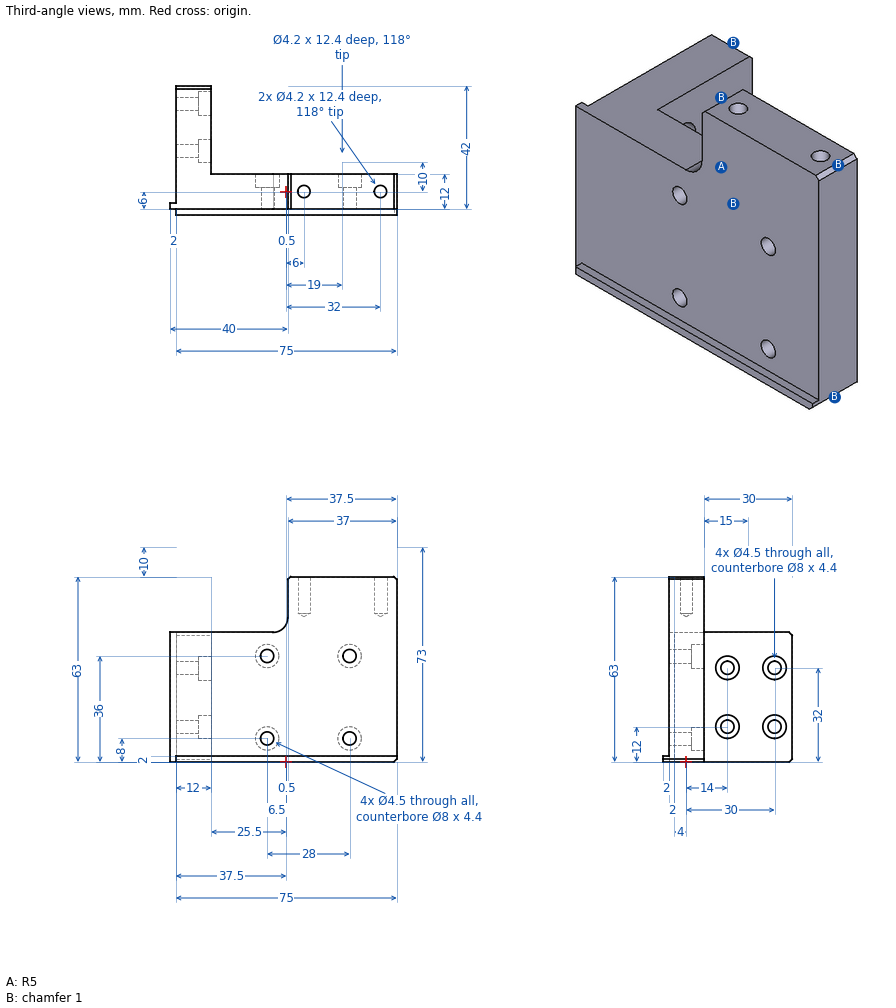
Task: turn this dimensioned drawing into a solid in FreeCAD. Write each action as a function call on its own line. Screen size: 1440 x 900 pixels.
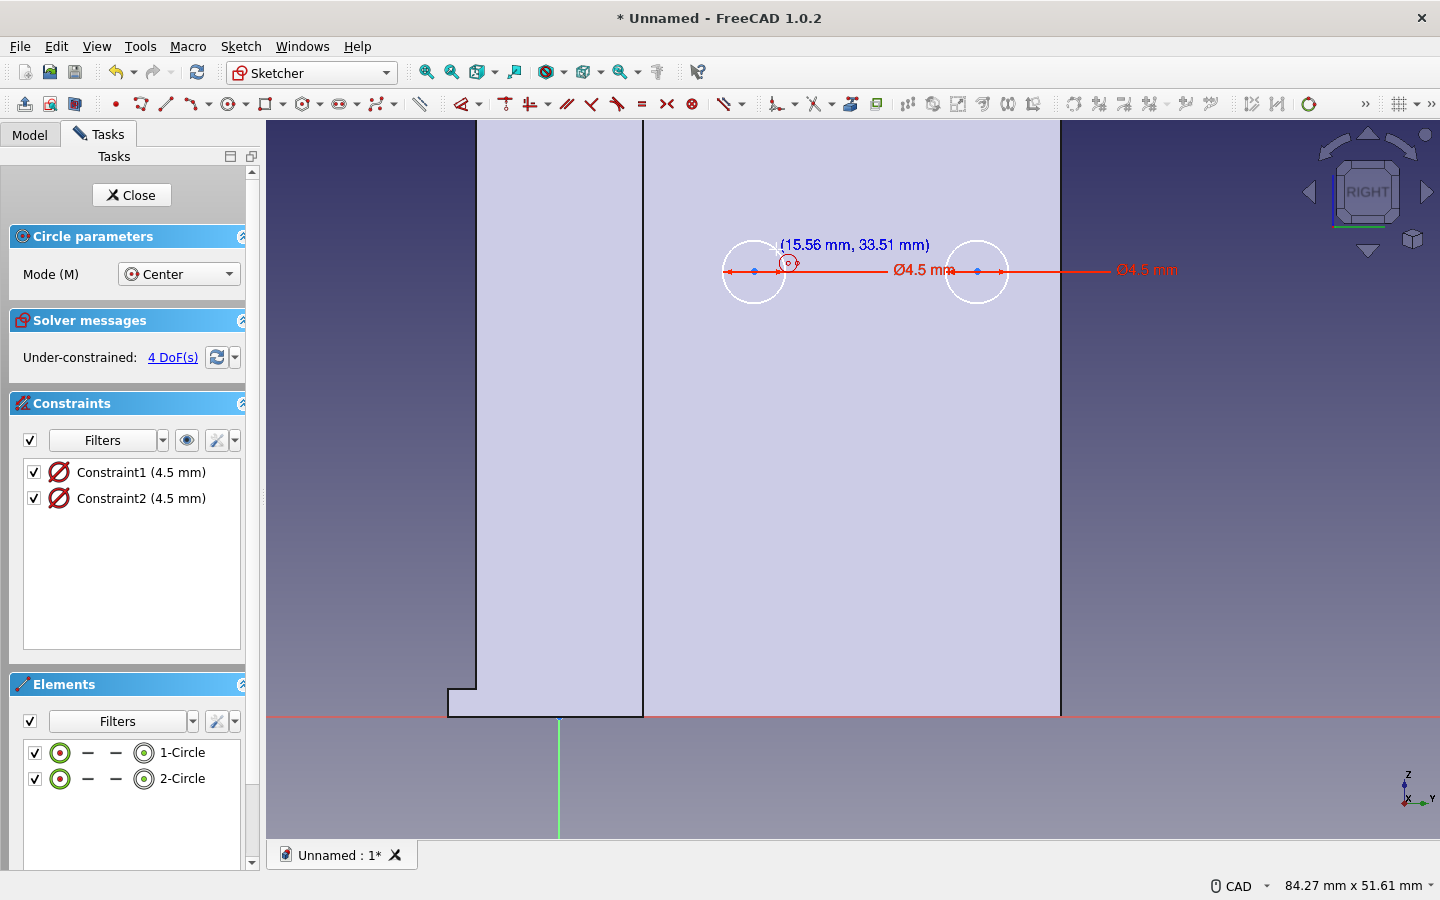
click(754, 550)
move(776, 527)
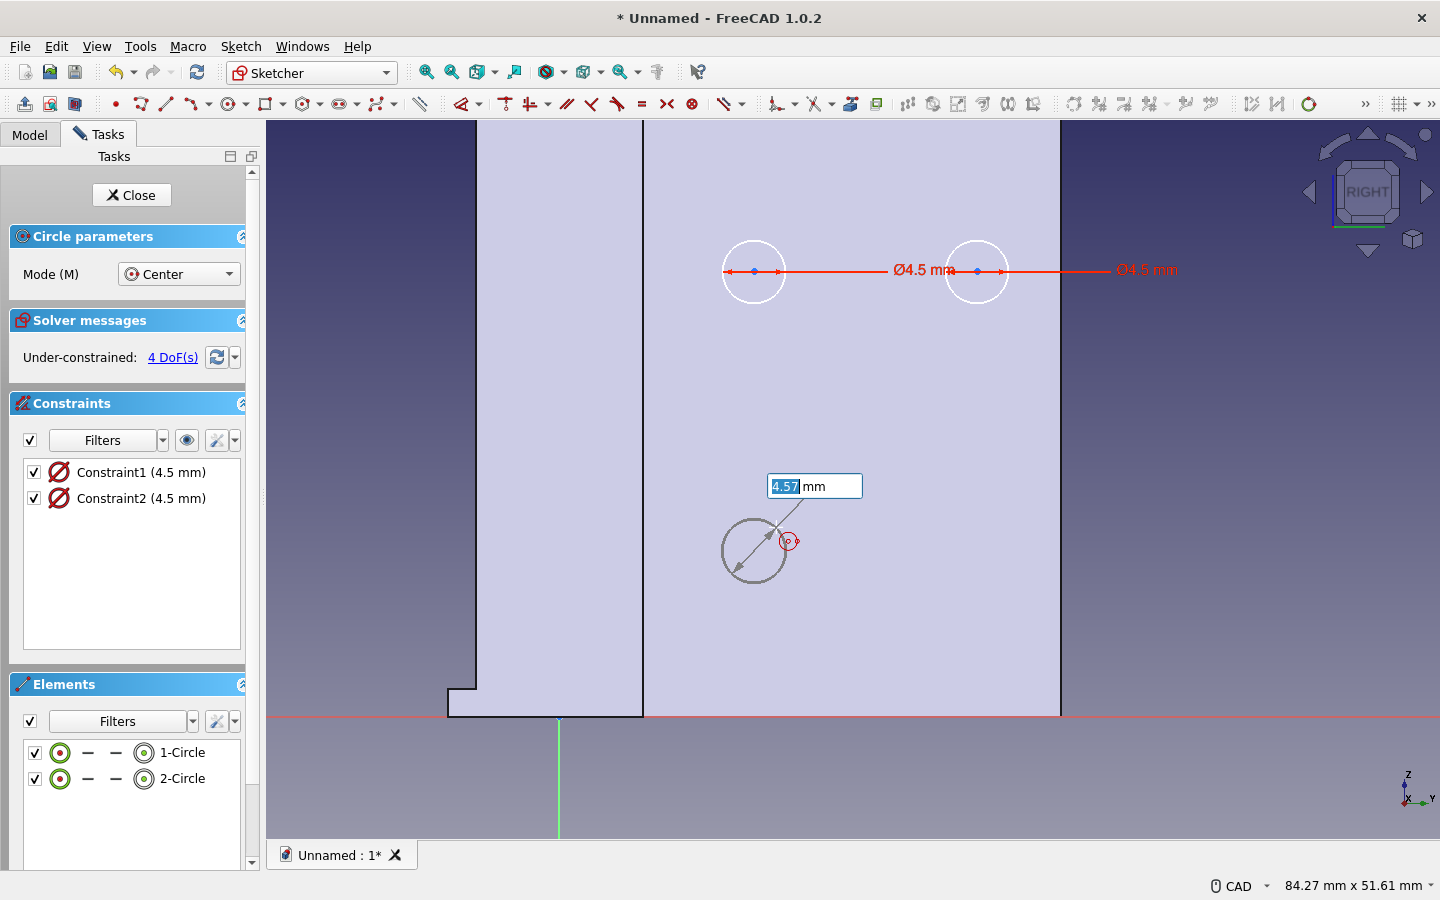
text(4.5)
key(Return)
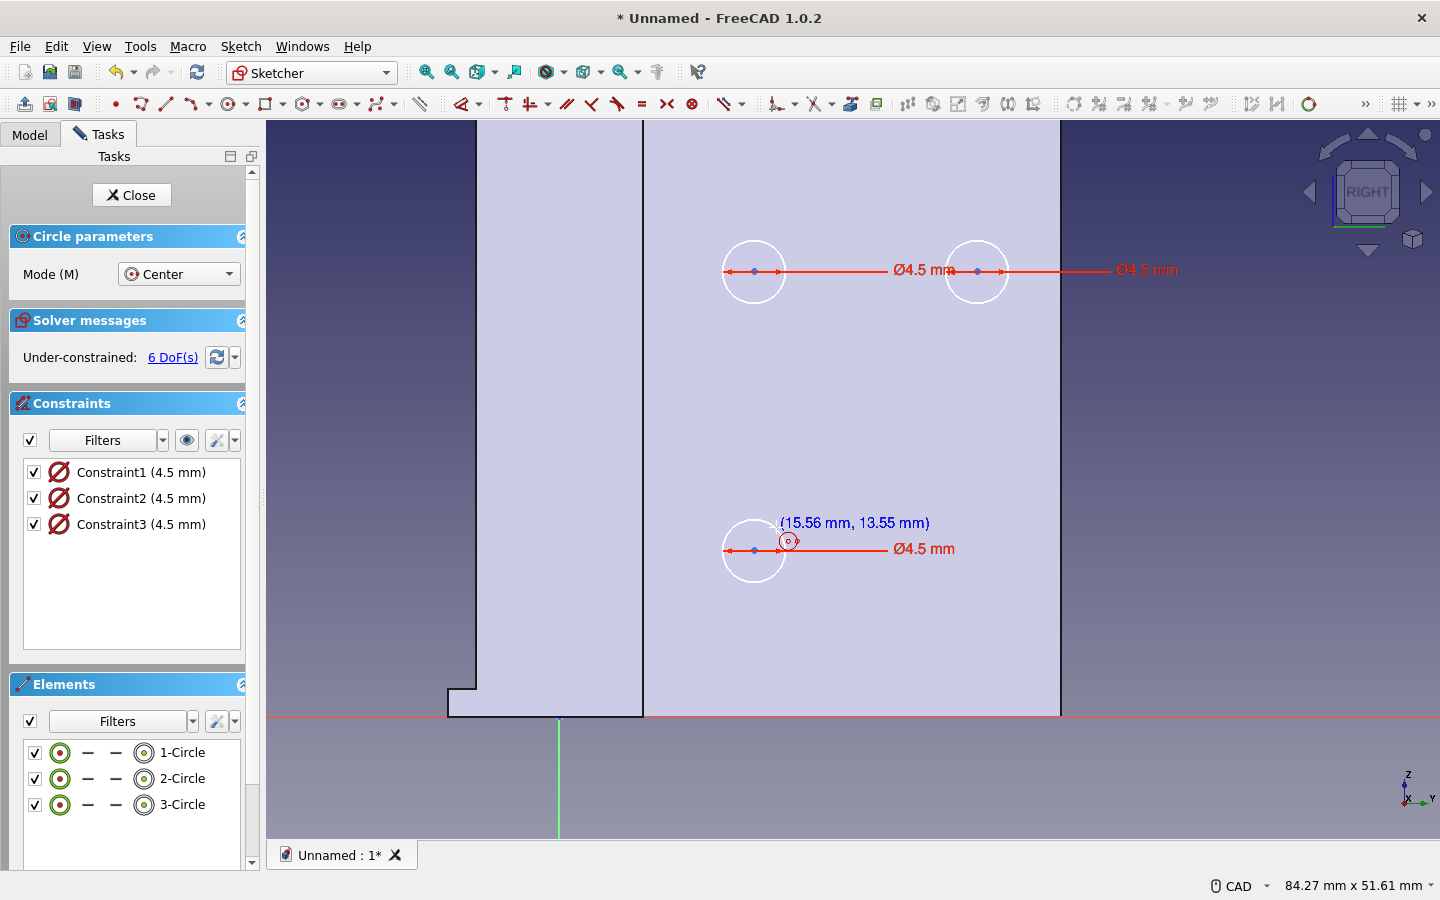
click(977, 550)
move(999, 527)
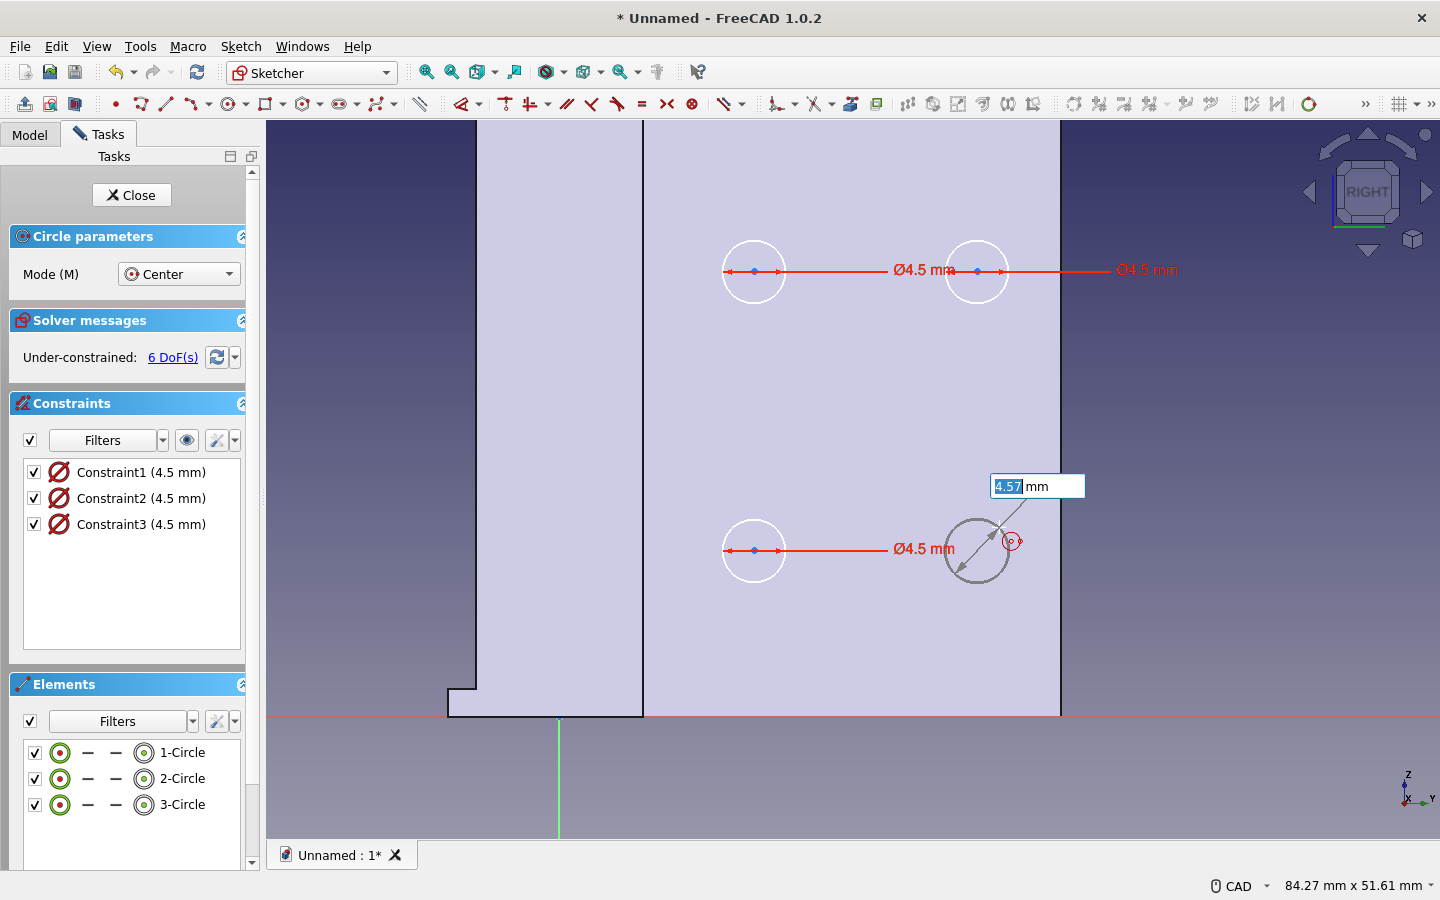
text(4.5)
key(Return)
key(Escape)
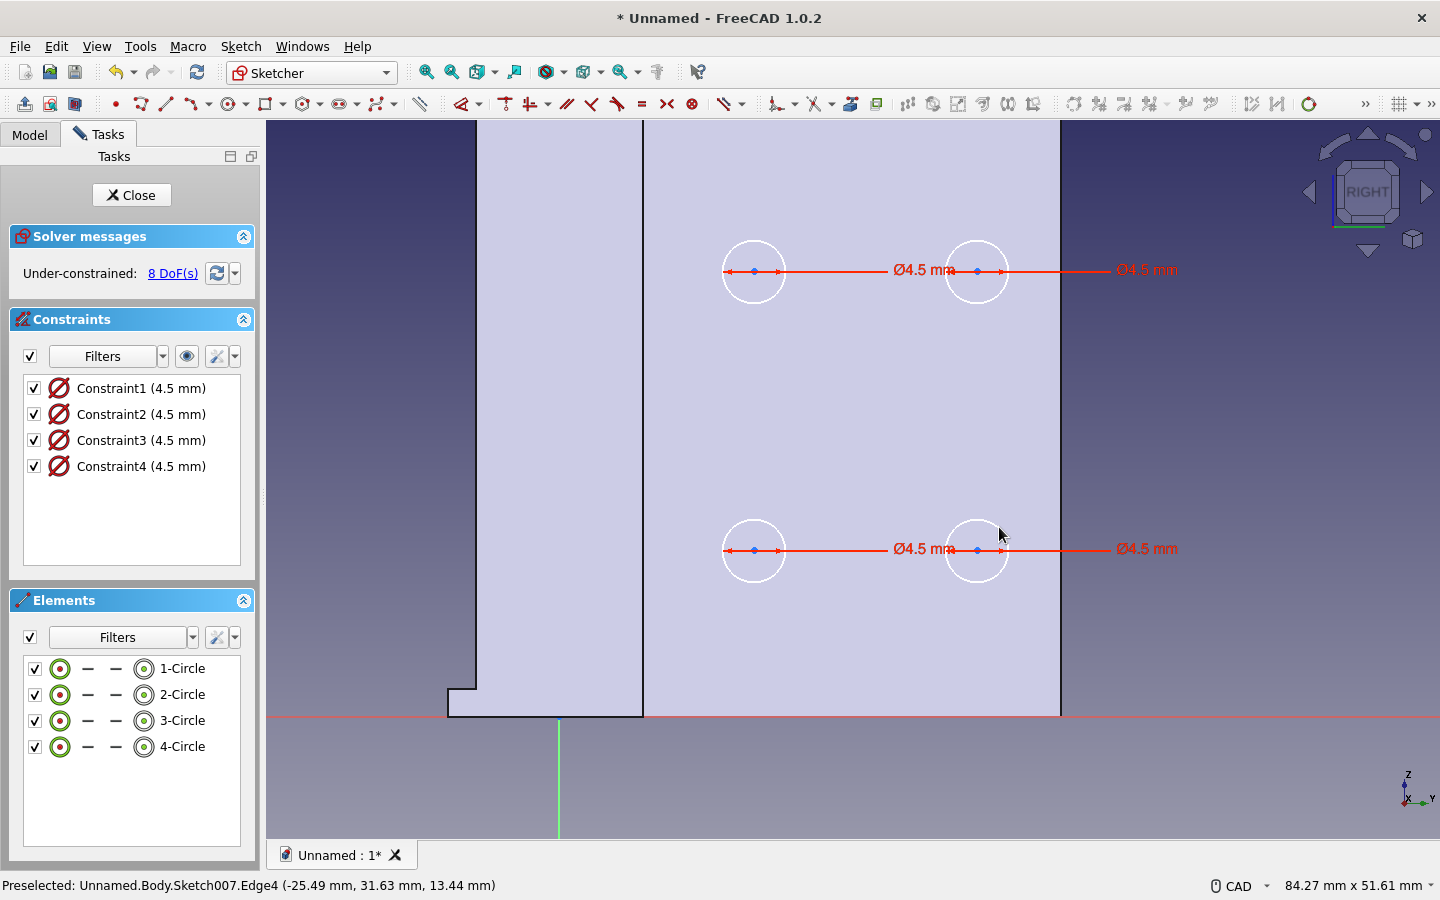
click(977, 272)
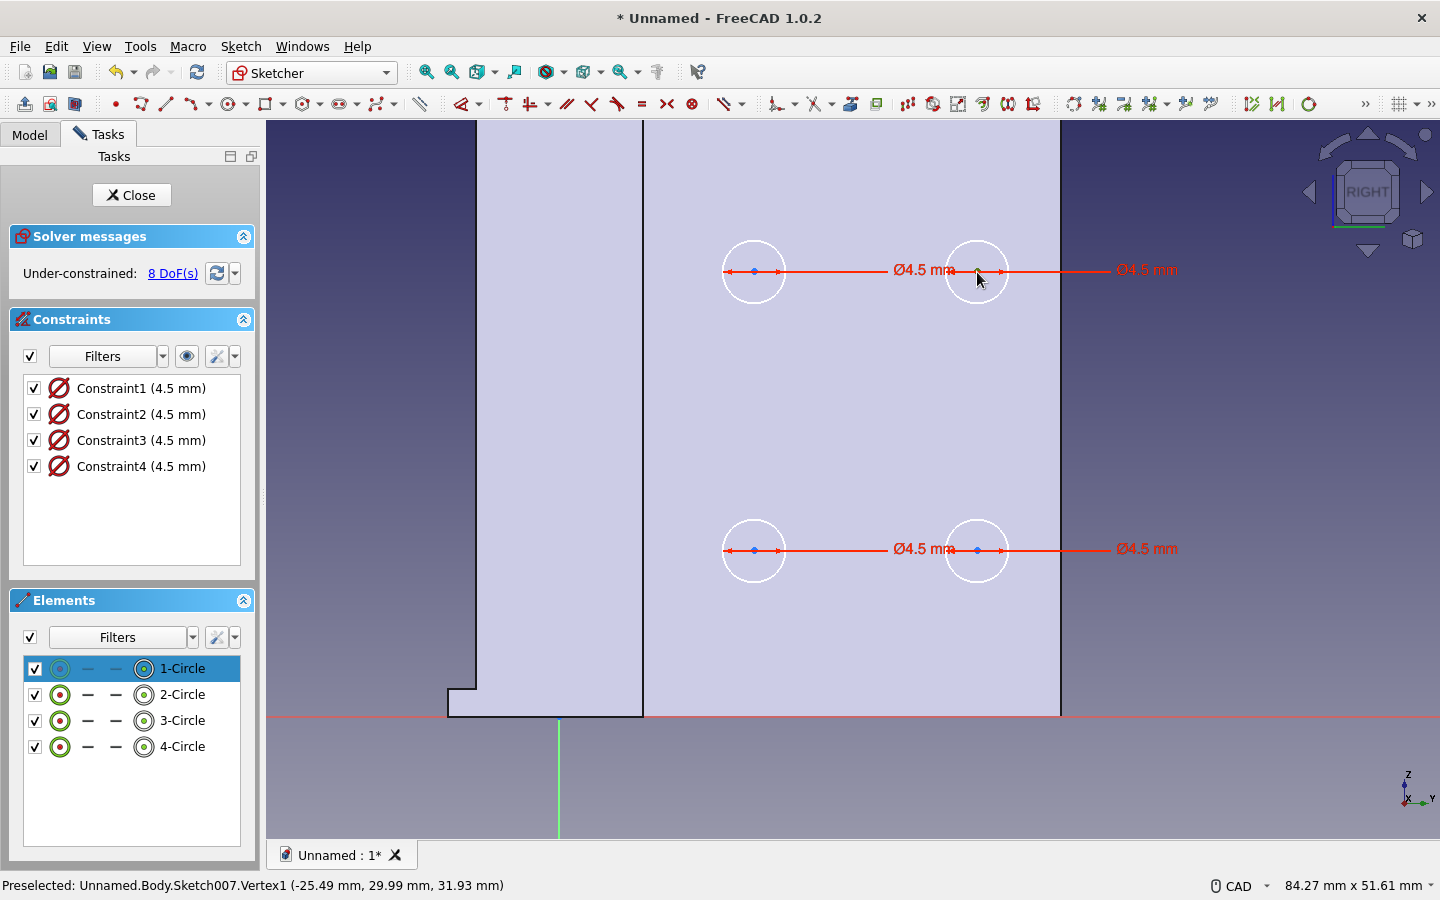
click(754, 272)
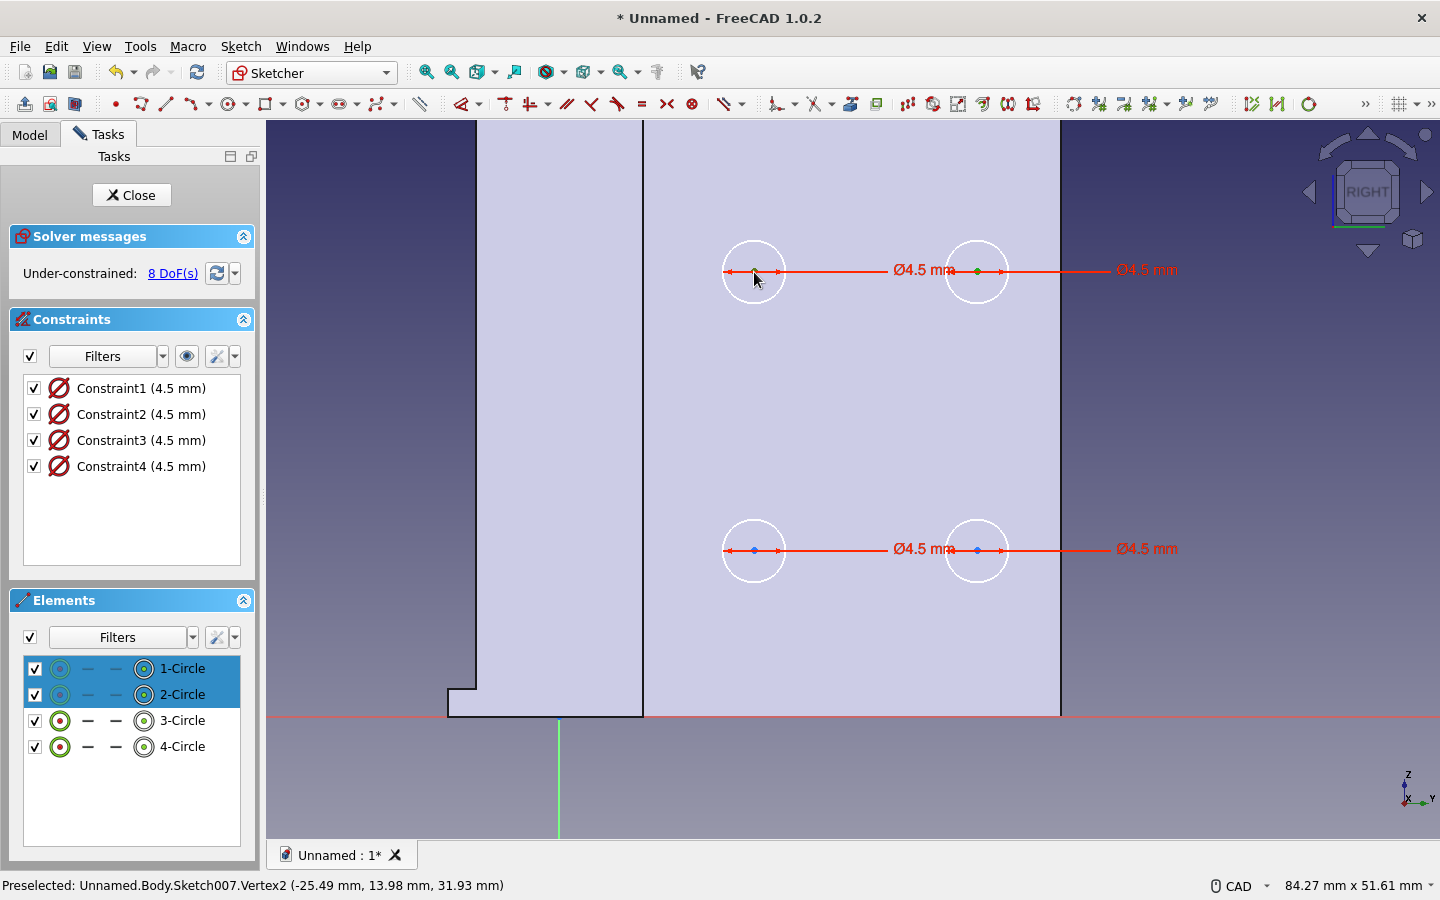
click(548, 104)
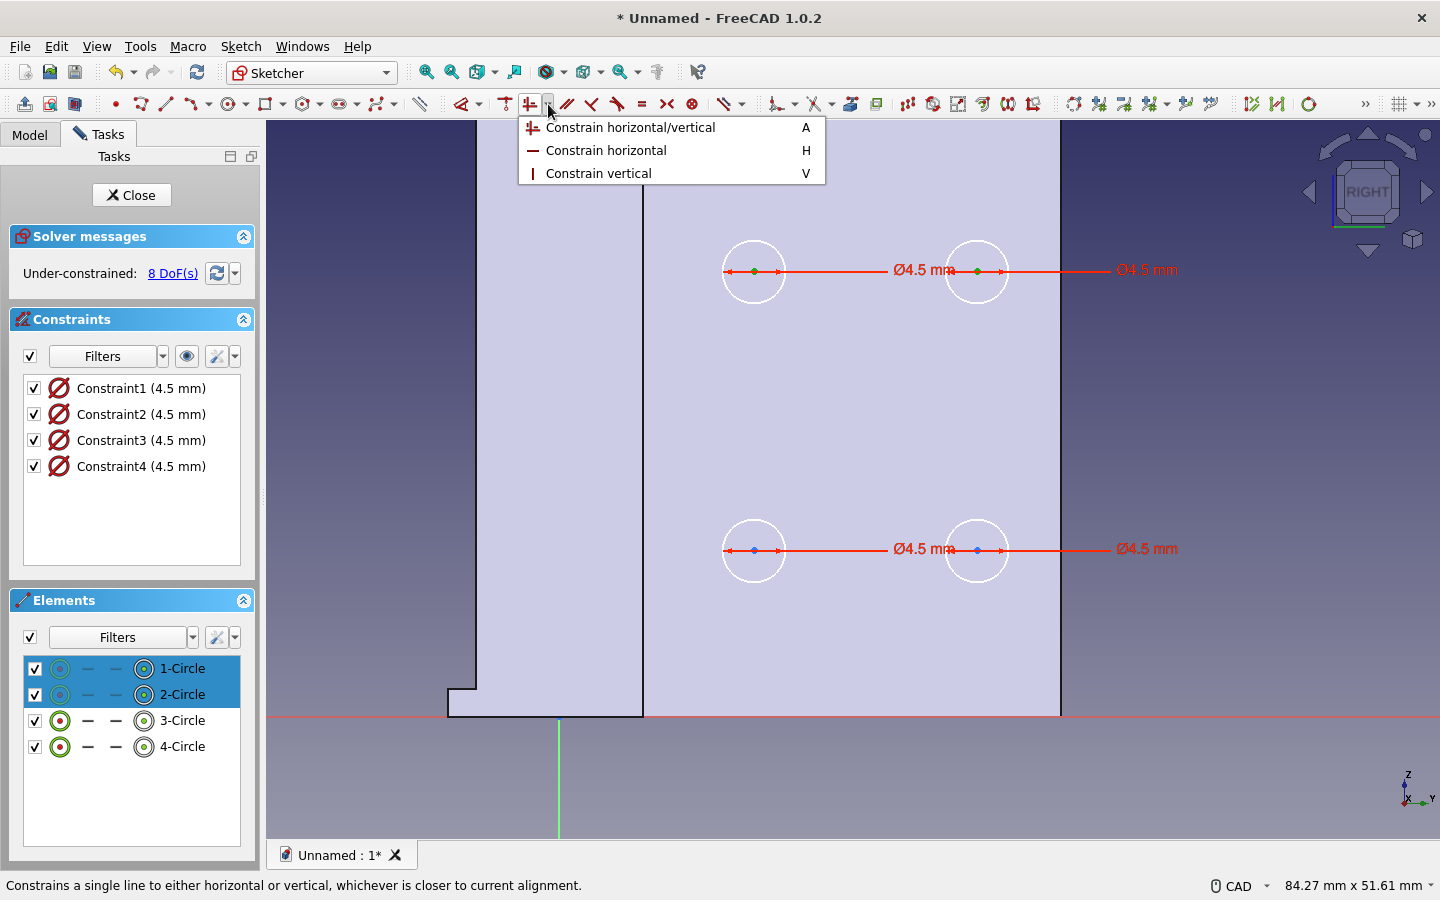
click(672, 150)